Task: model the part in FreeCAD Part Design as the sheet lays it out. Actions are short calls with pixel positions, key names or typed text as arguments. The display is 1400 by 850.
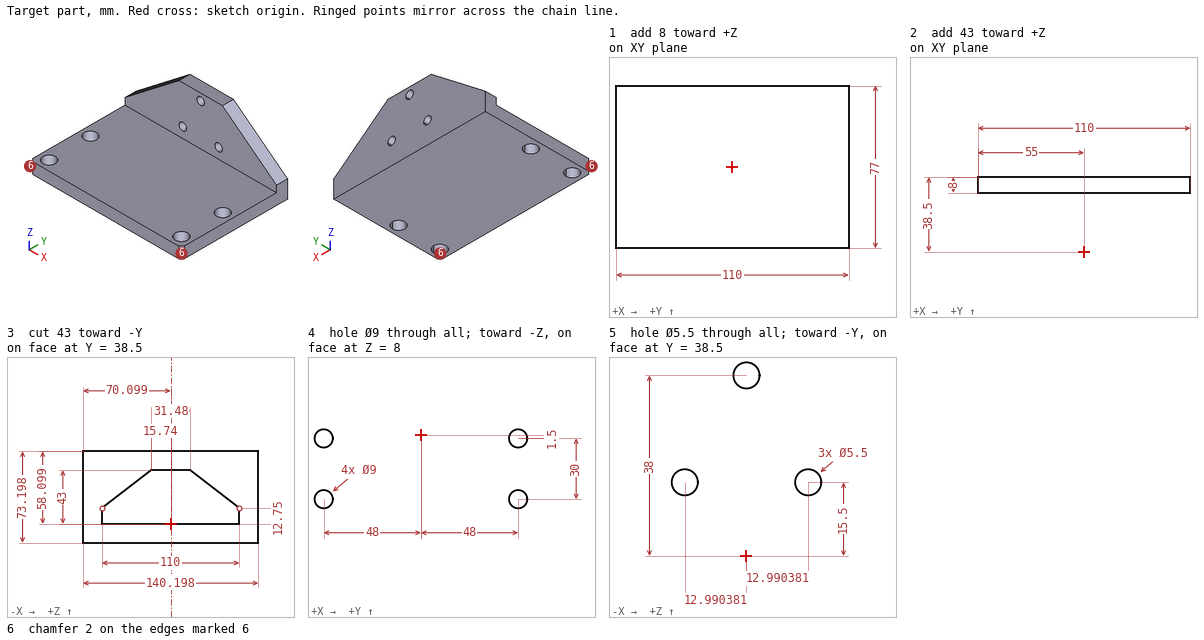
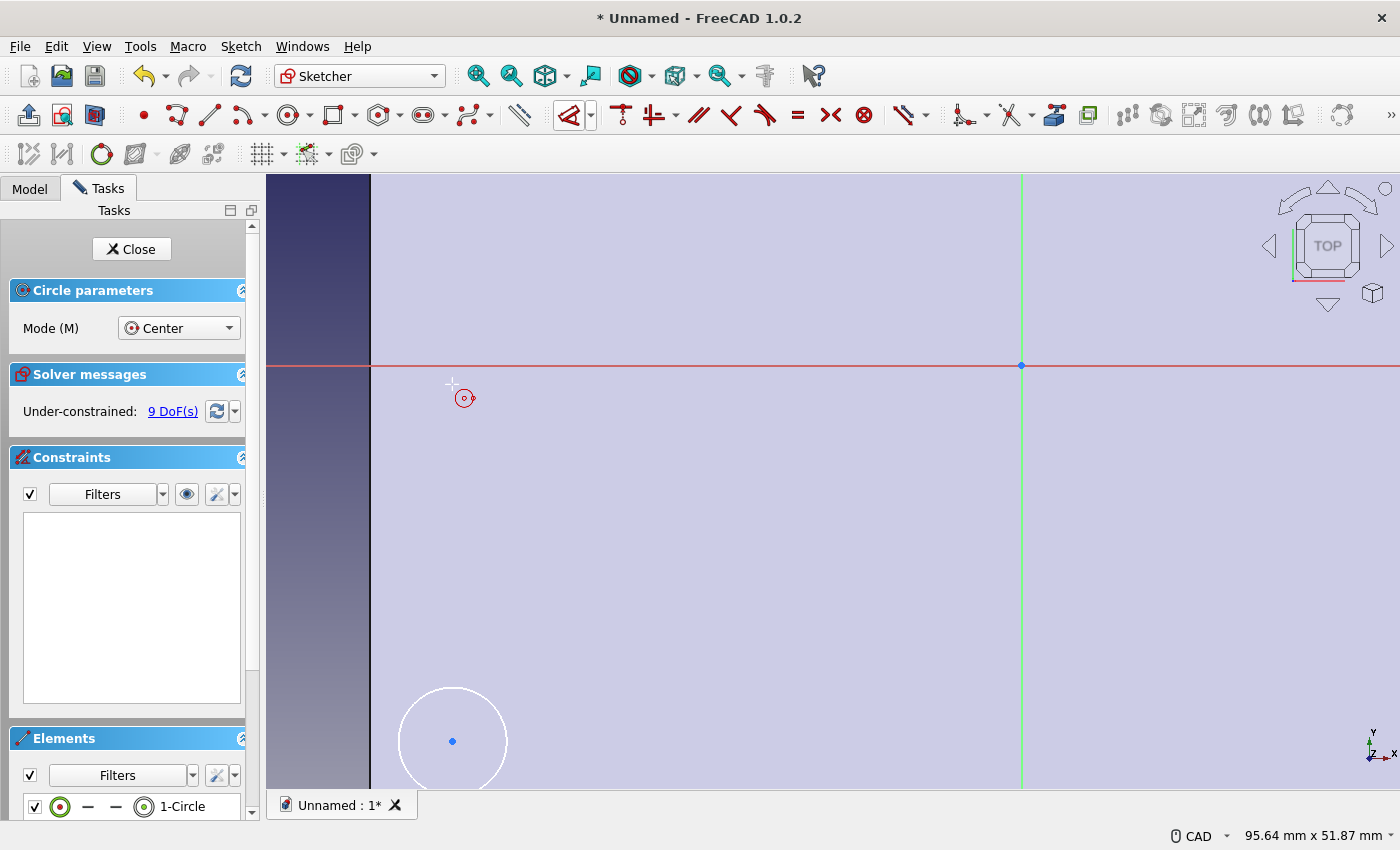
click(453, 383)
click(490, 346)
key(Escape)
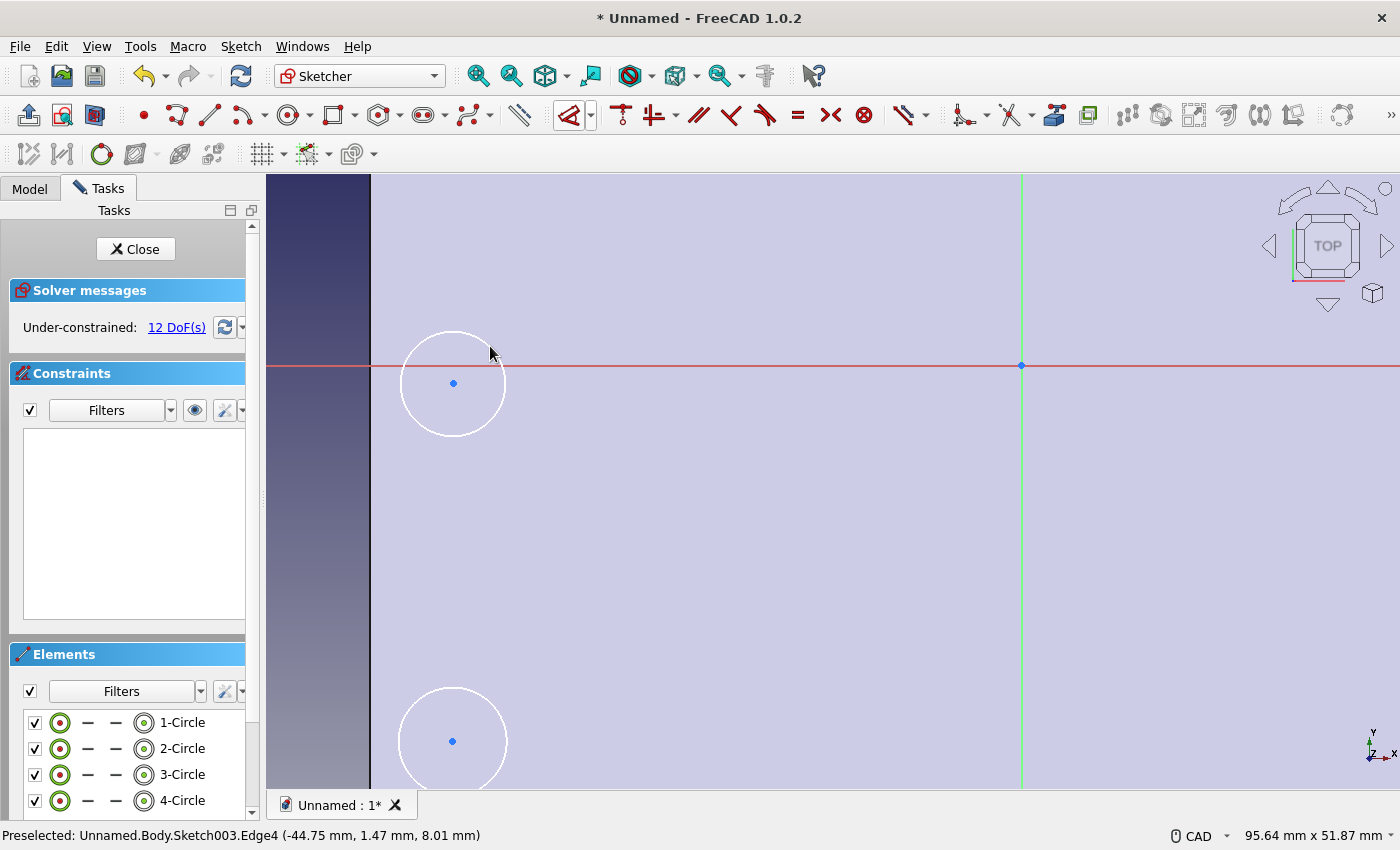
click(491, 703)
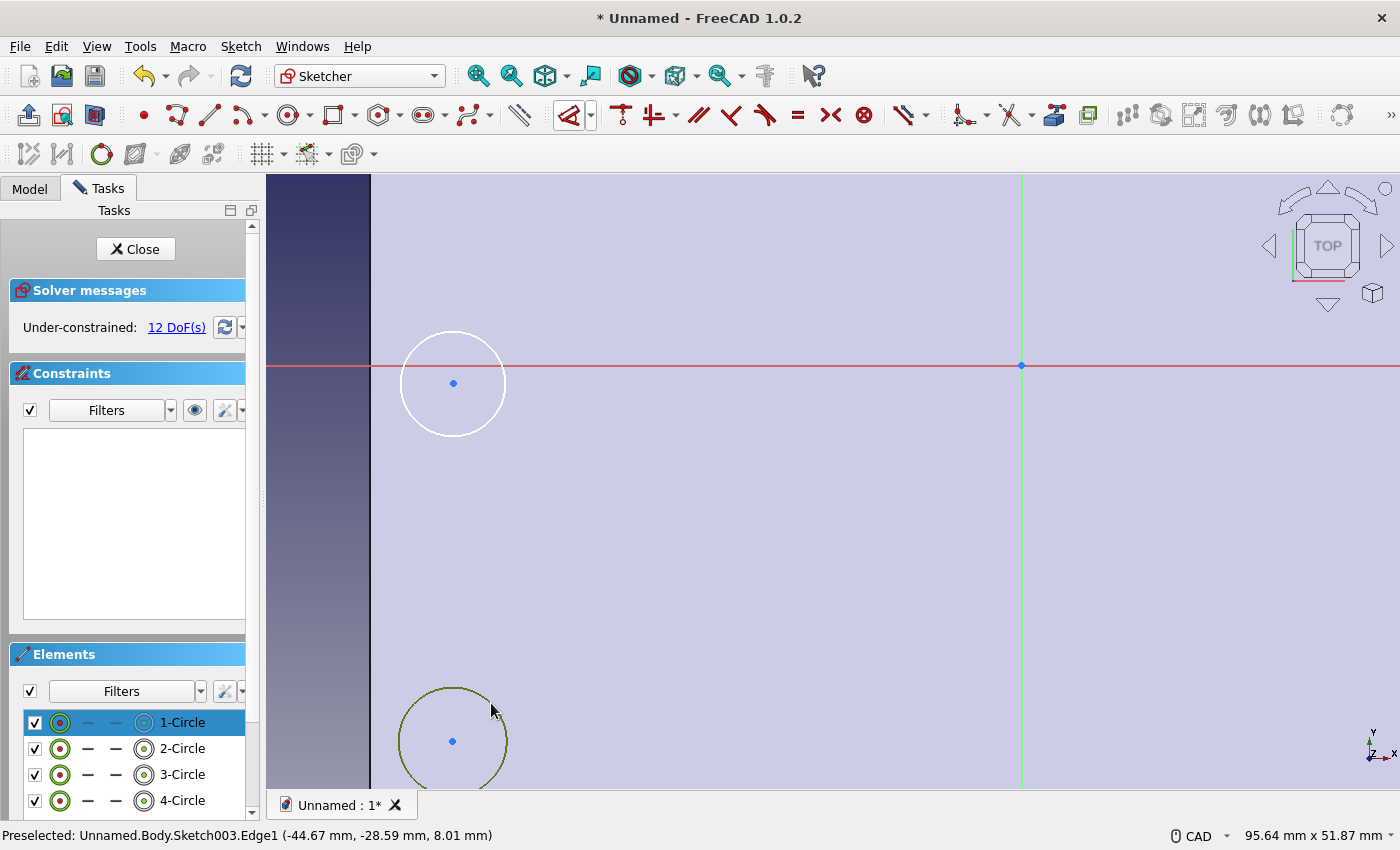
scroll(452, 384, down, 3)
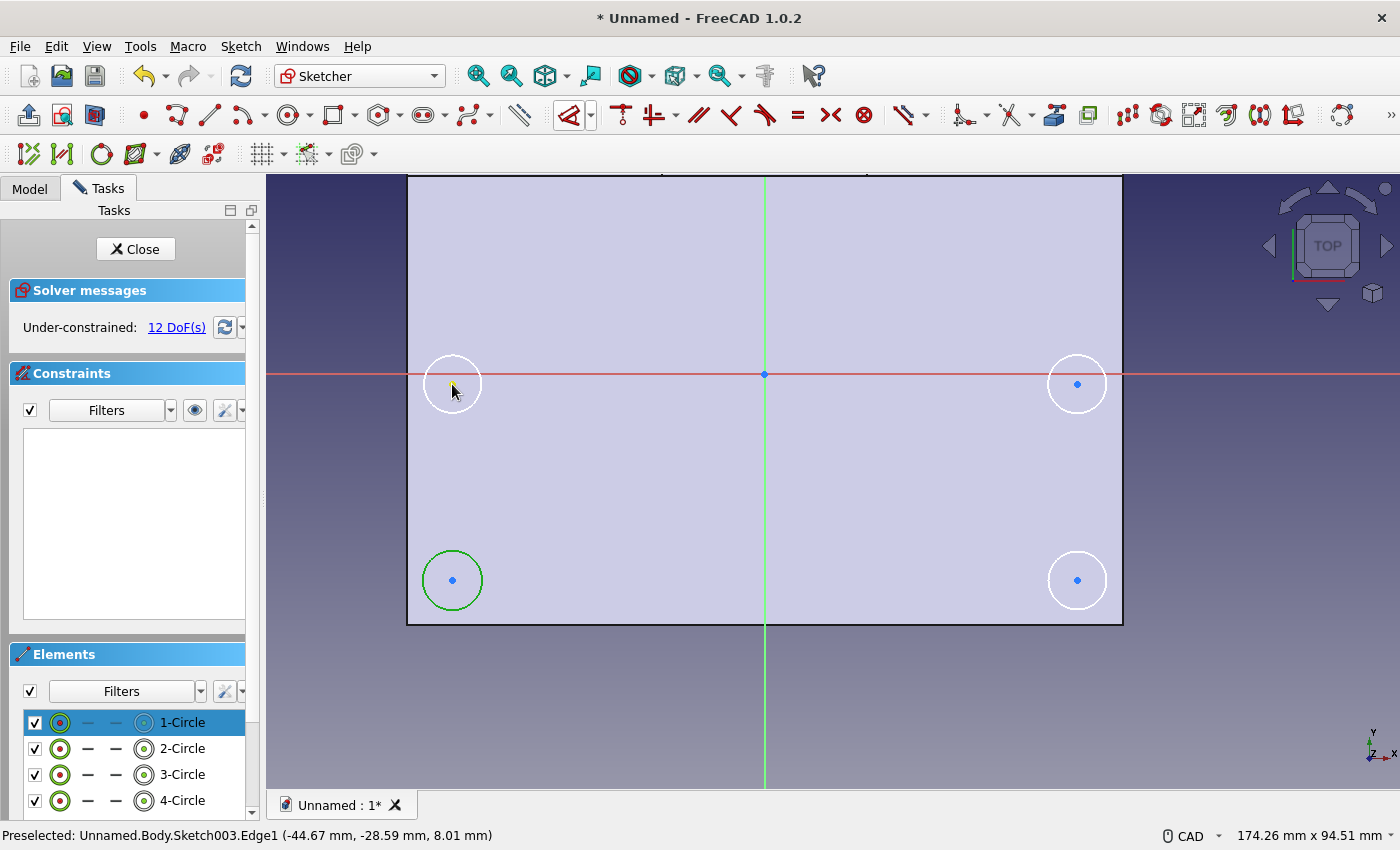
click(1098, 560)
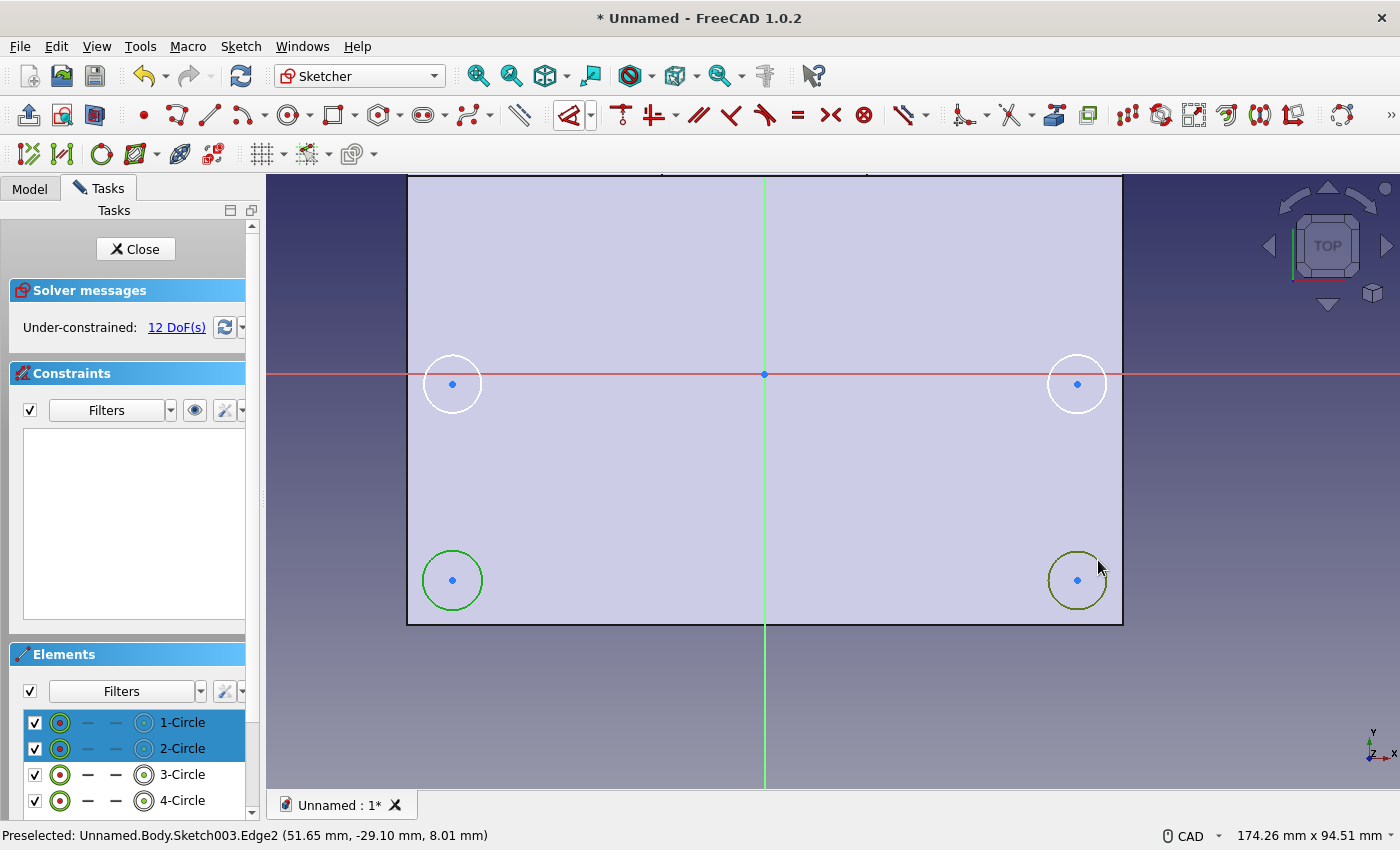
scroll(1098, 364, up, 2)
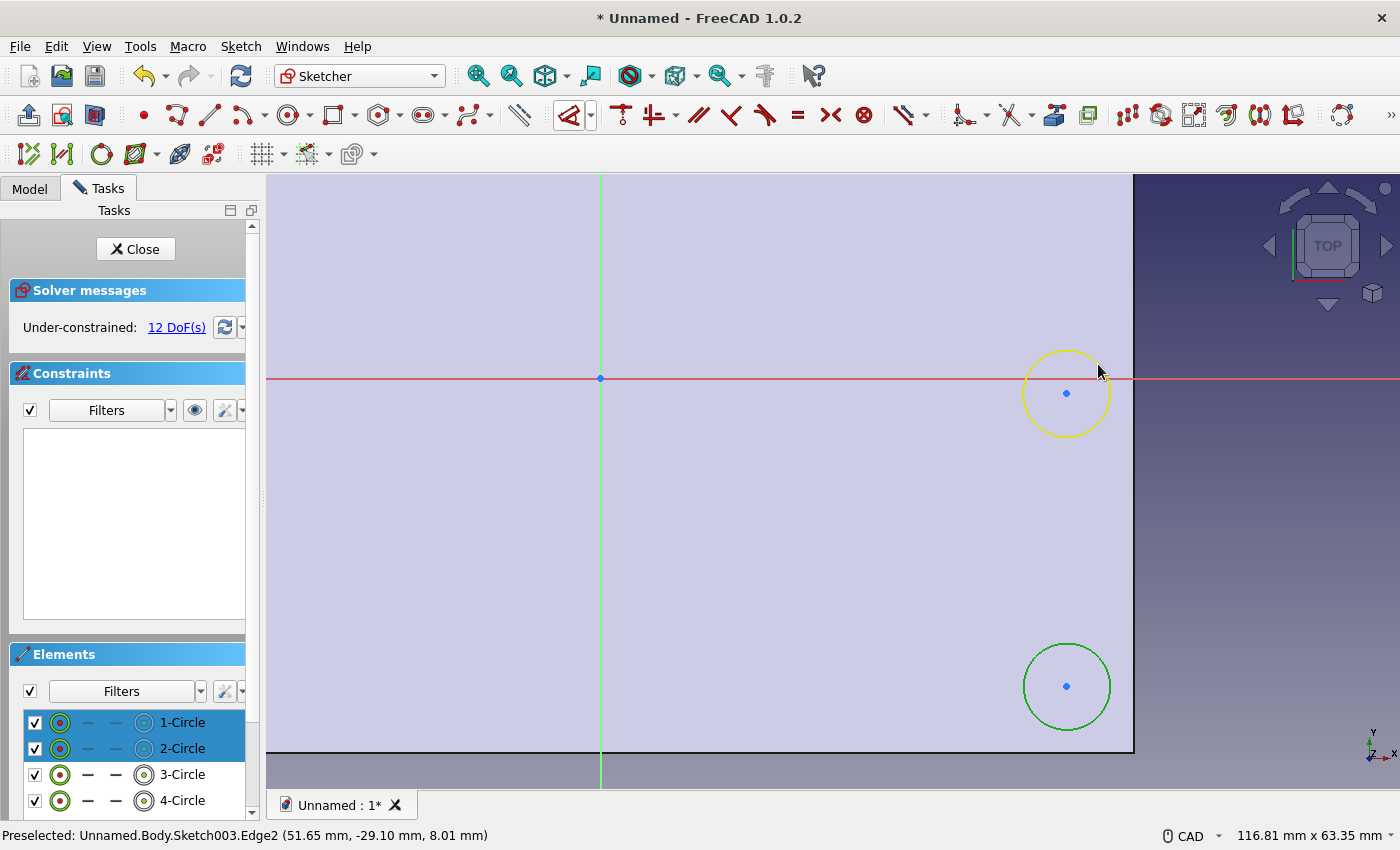
click(1097, 363)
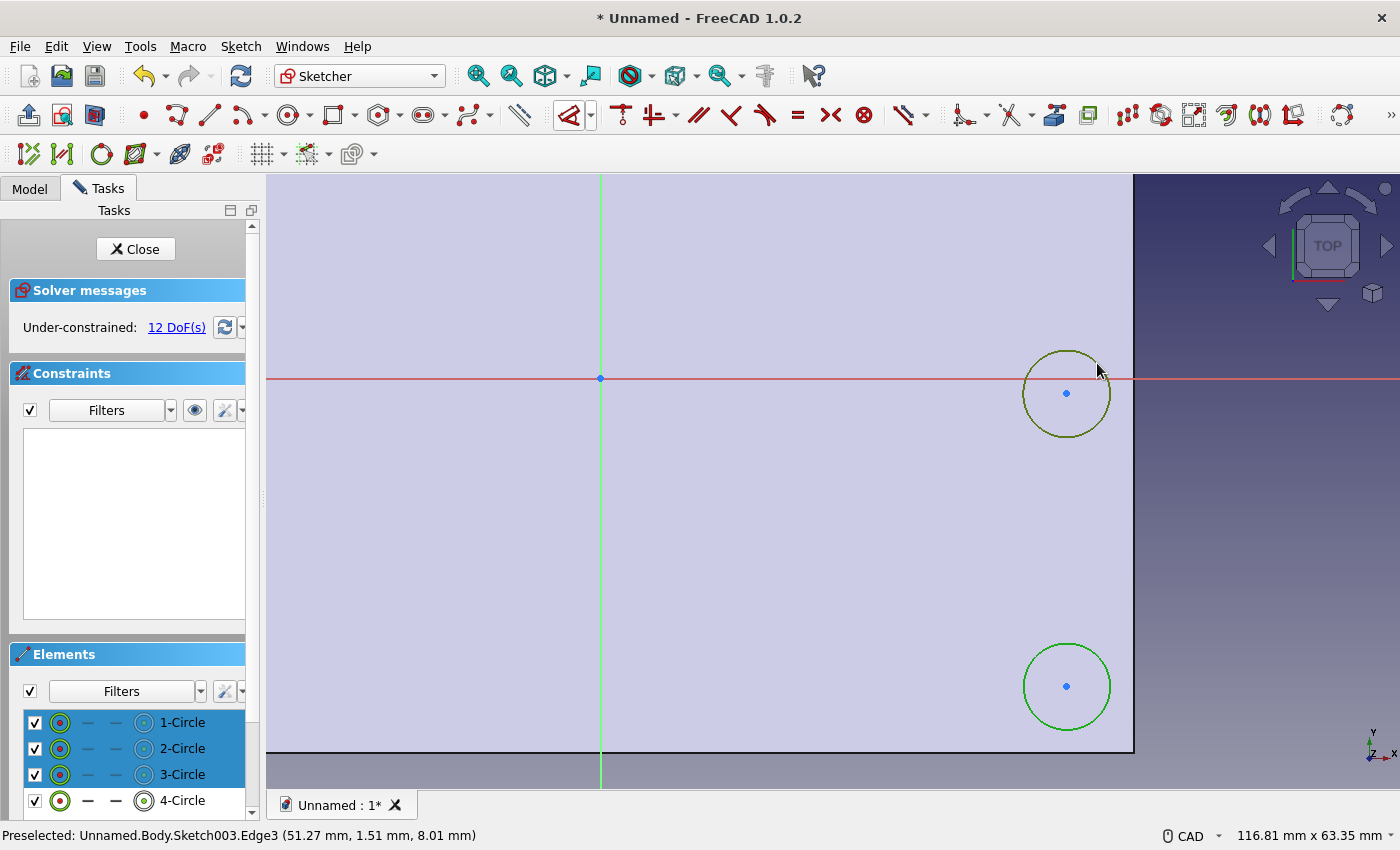
scroll(1098, 364, down, 2)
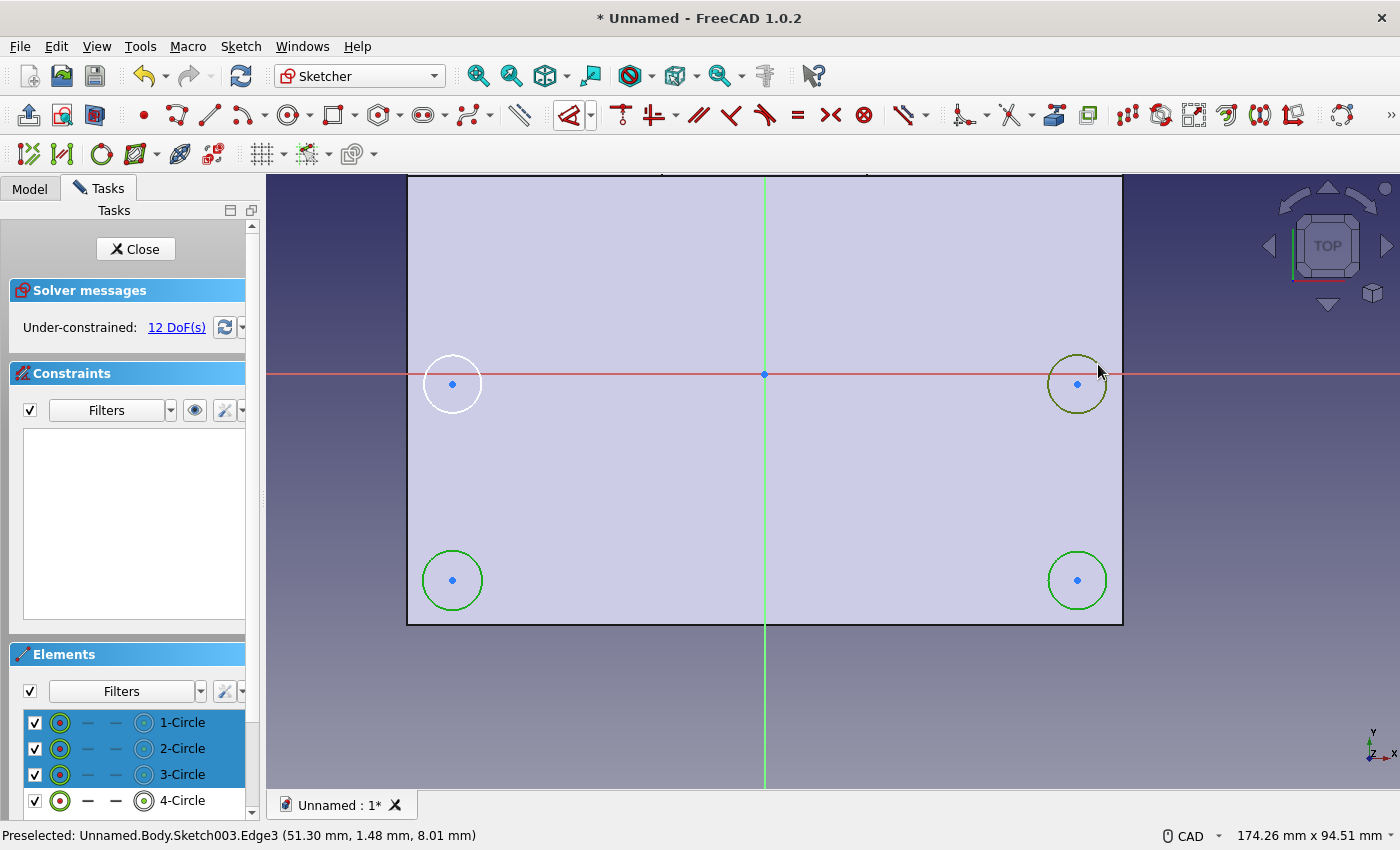
scroll(473, 364, up, 2)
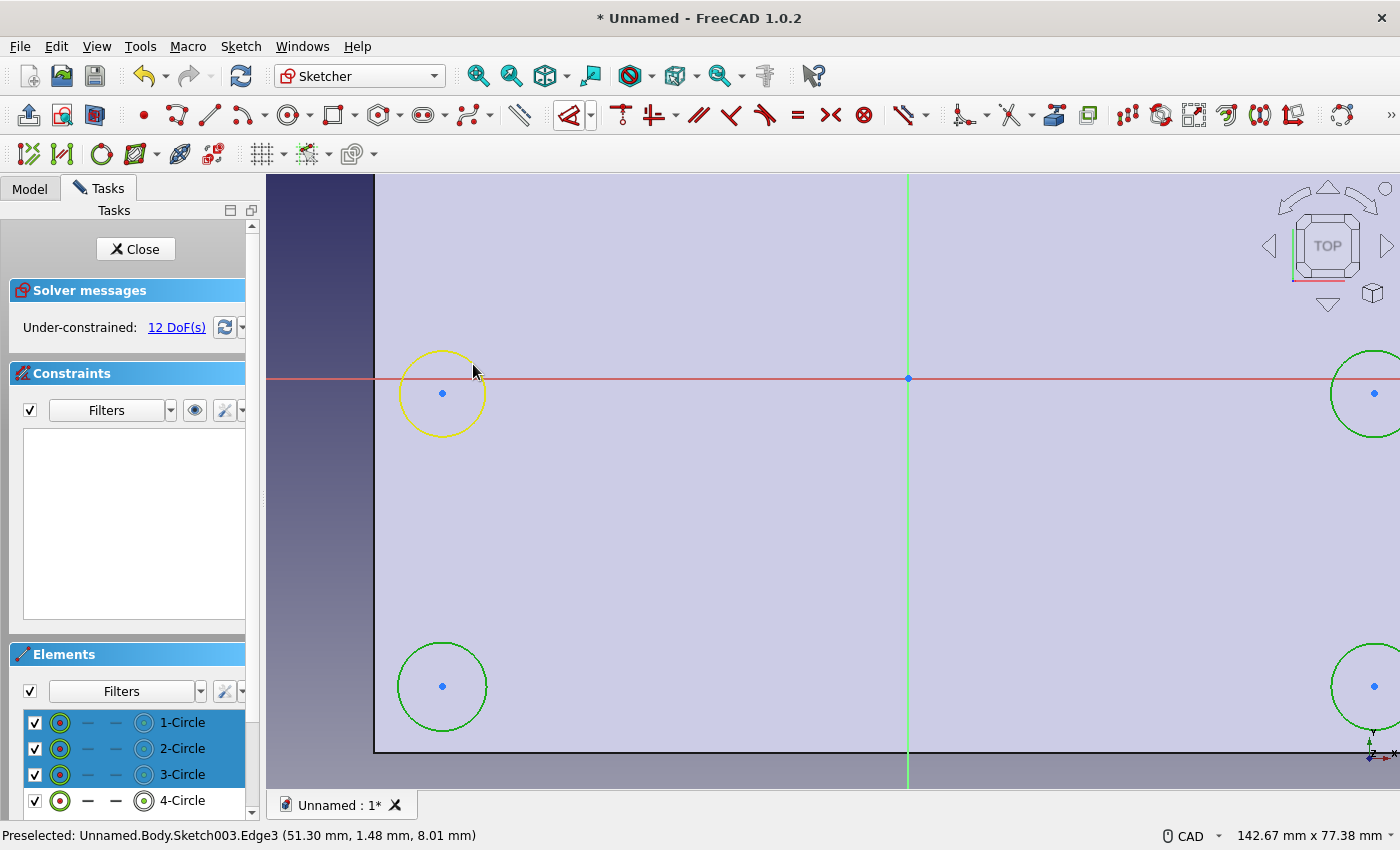
click(473, 364)